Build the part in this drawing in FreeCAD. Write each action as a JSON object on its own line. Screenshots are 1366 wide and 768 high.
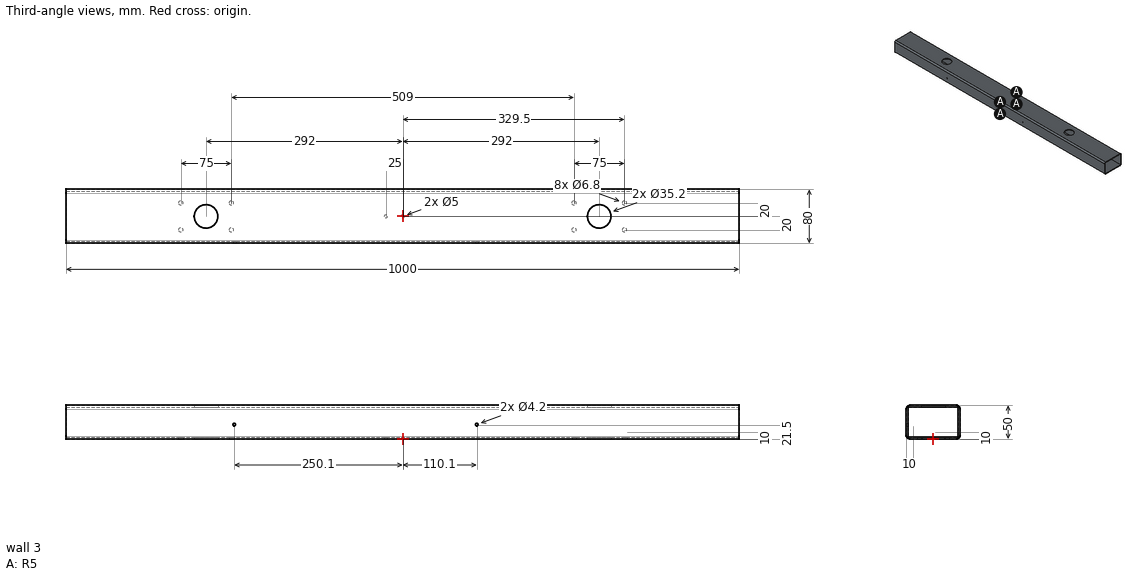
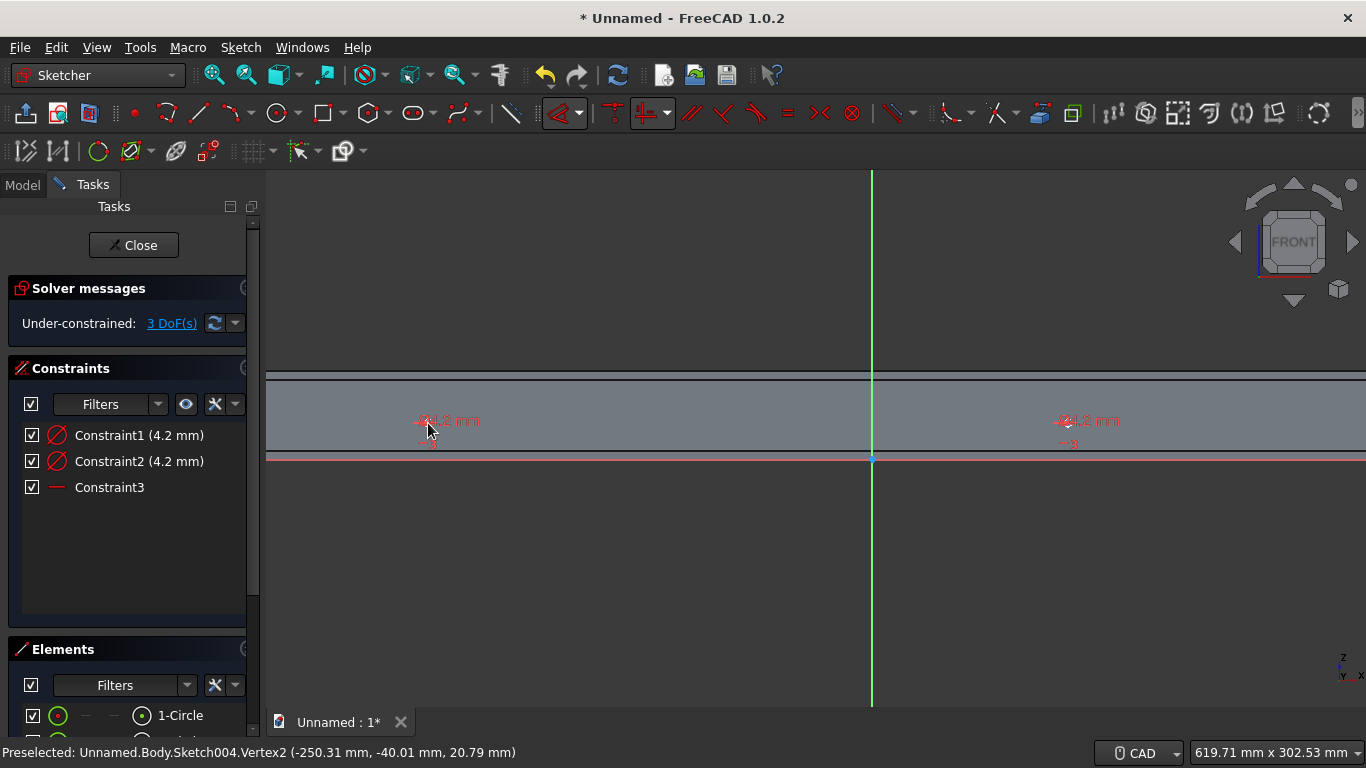
{"action": "left_click", "coordinate": [1068, 423]}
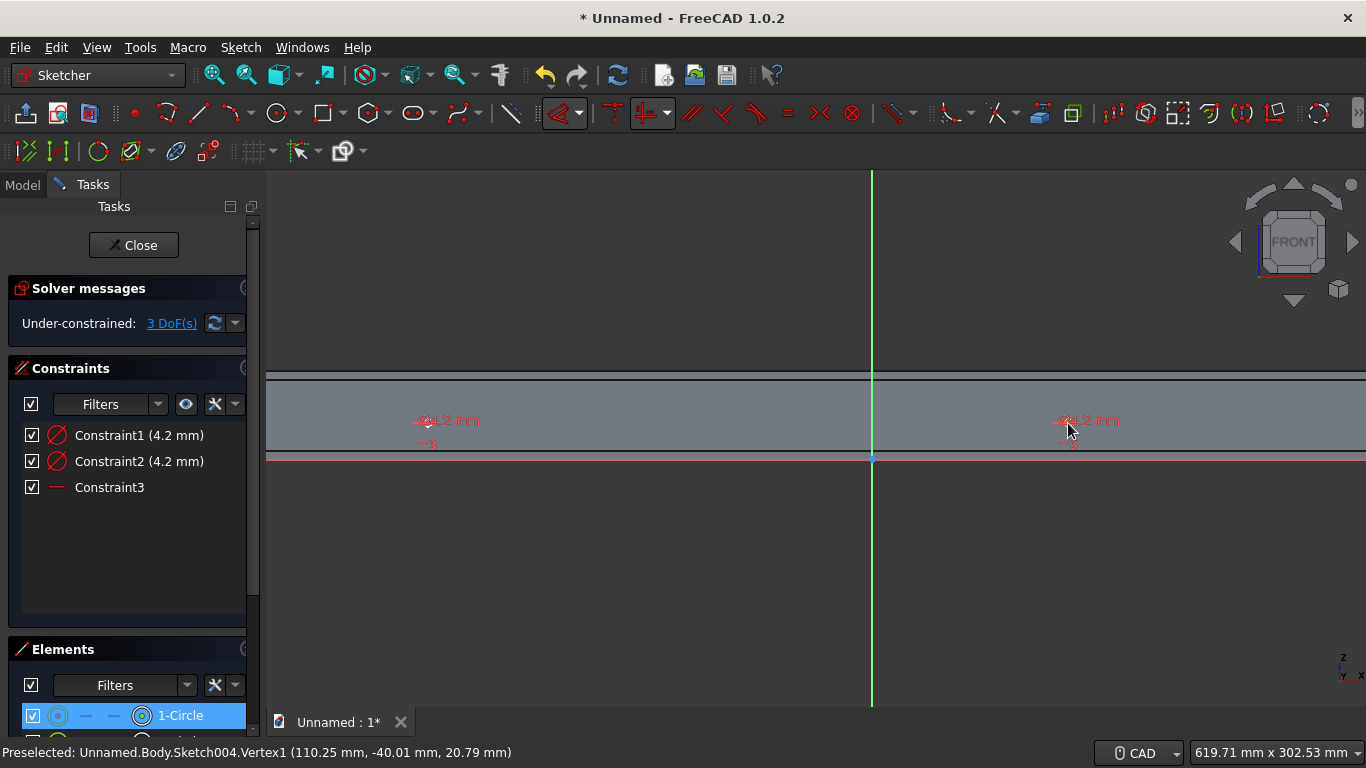
{"action": "left_click", "coordinate": [582, 114]}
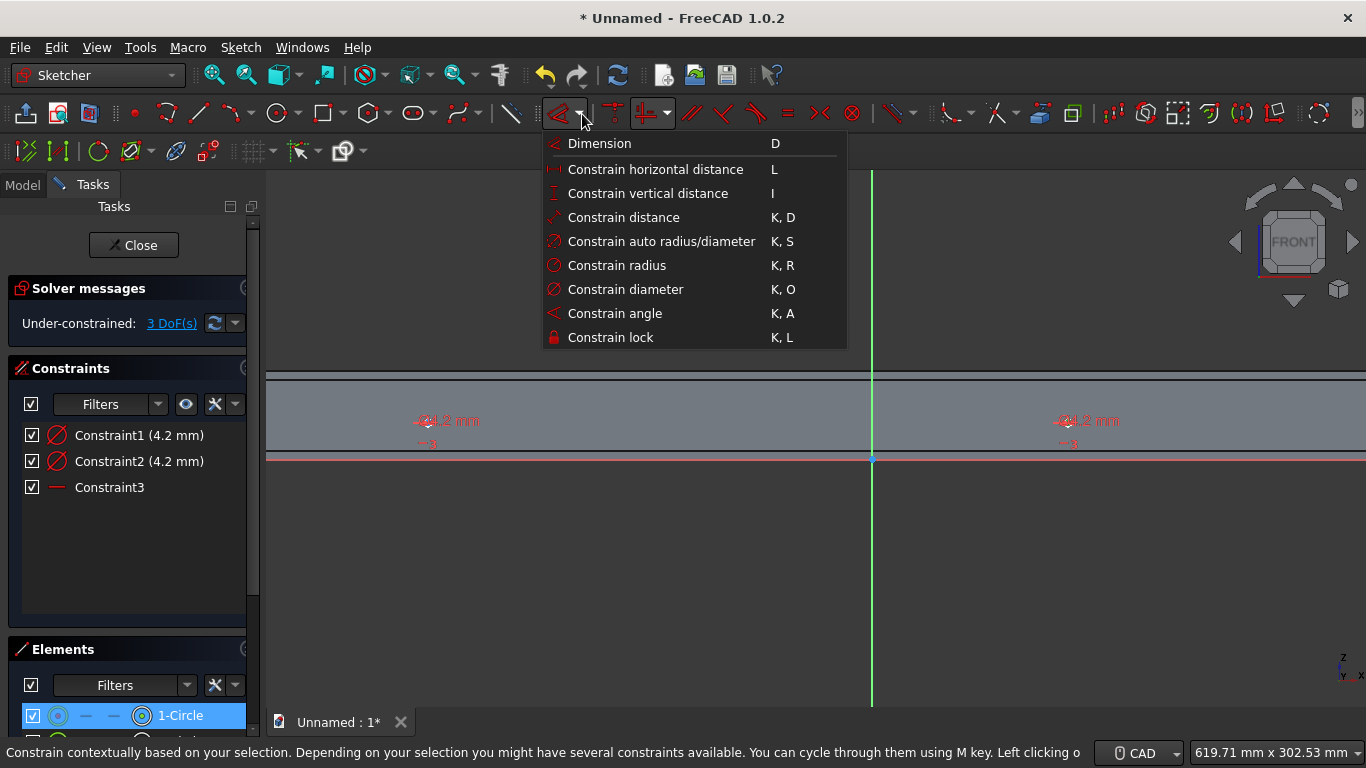
{"action": "left_click", "coordinate": [695, 193]}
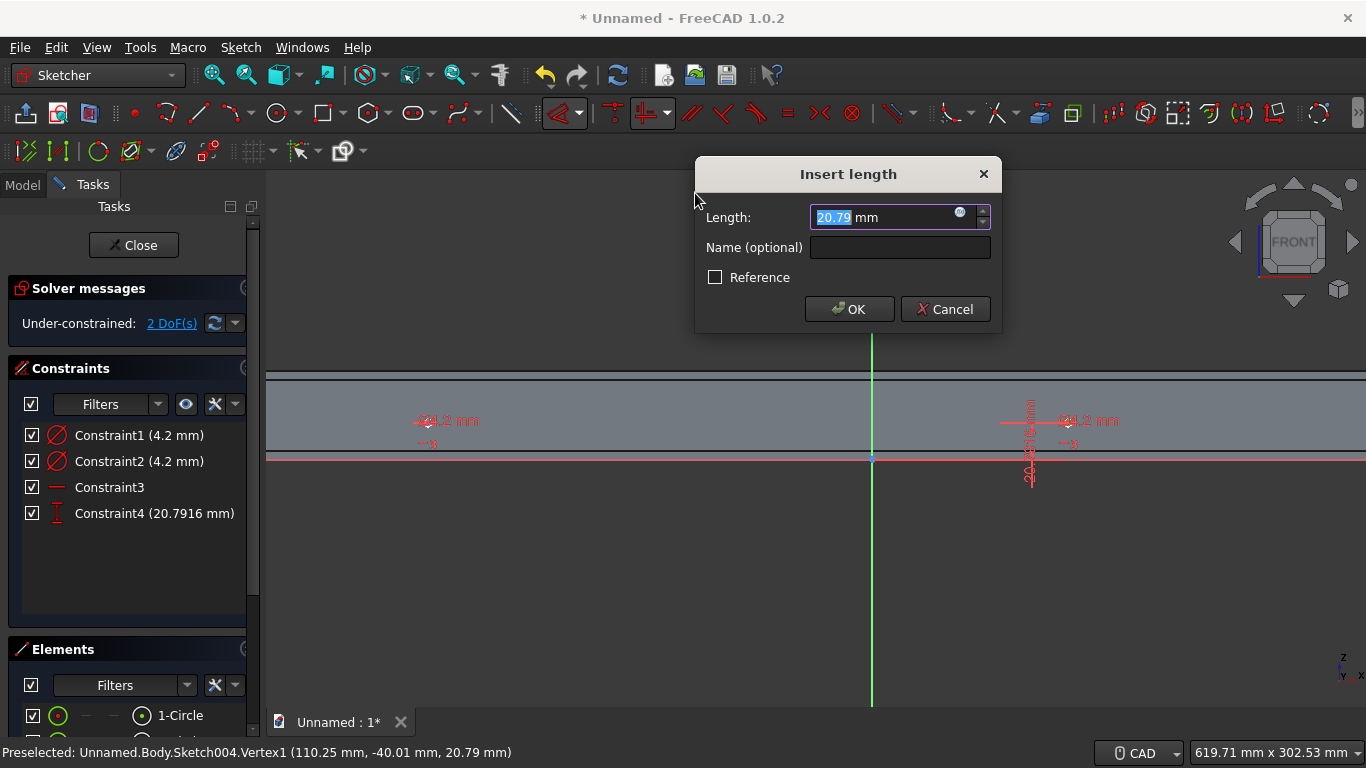
{"action": "type", "text": "21.5"}
{"action": "key", "text": "Return"}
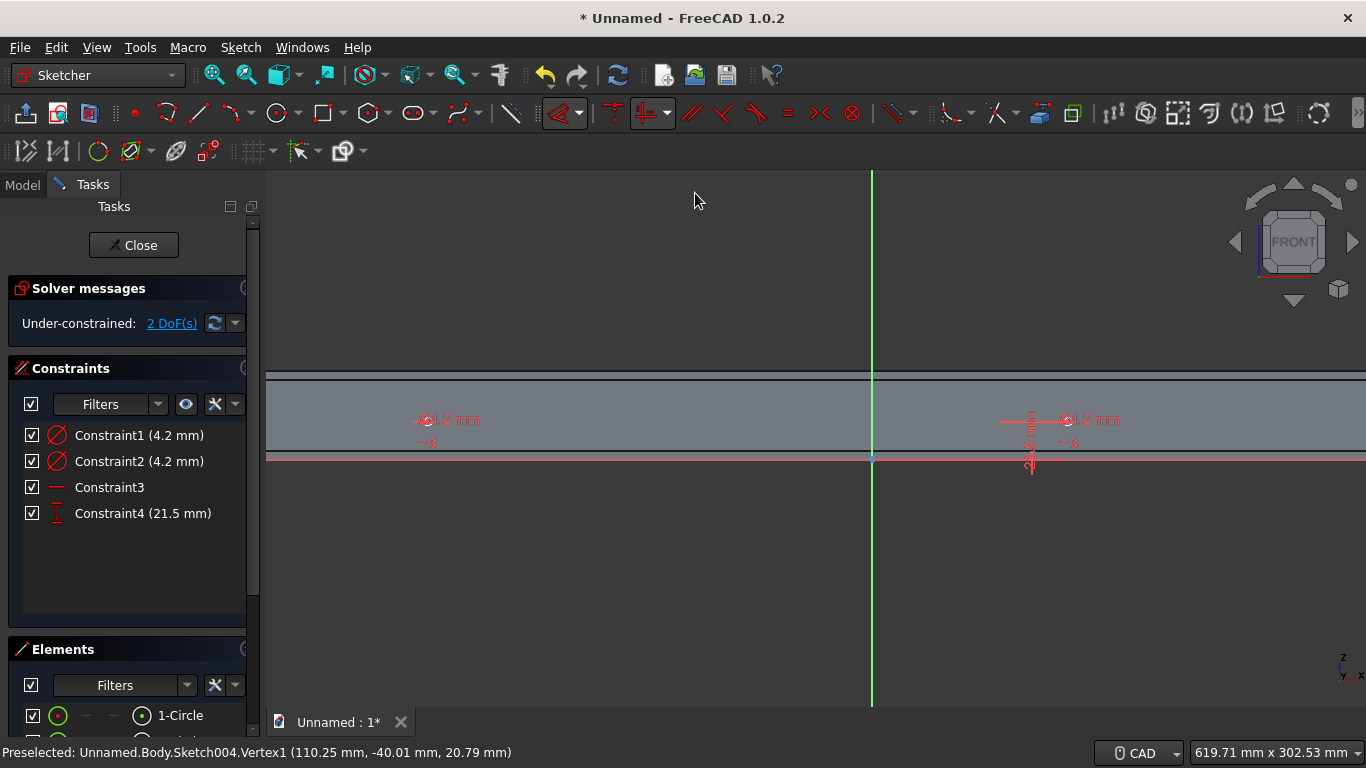
{"action": "left_click", "coordinate": [1068, 422]}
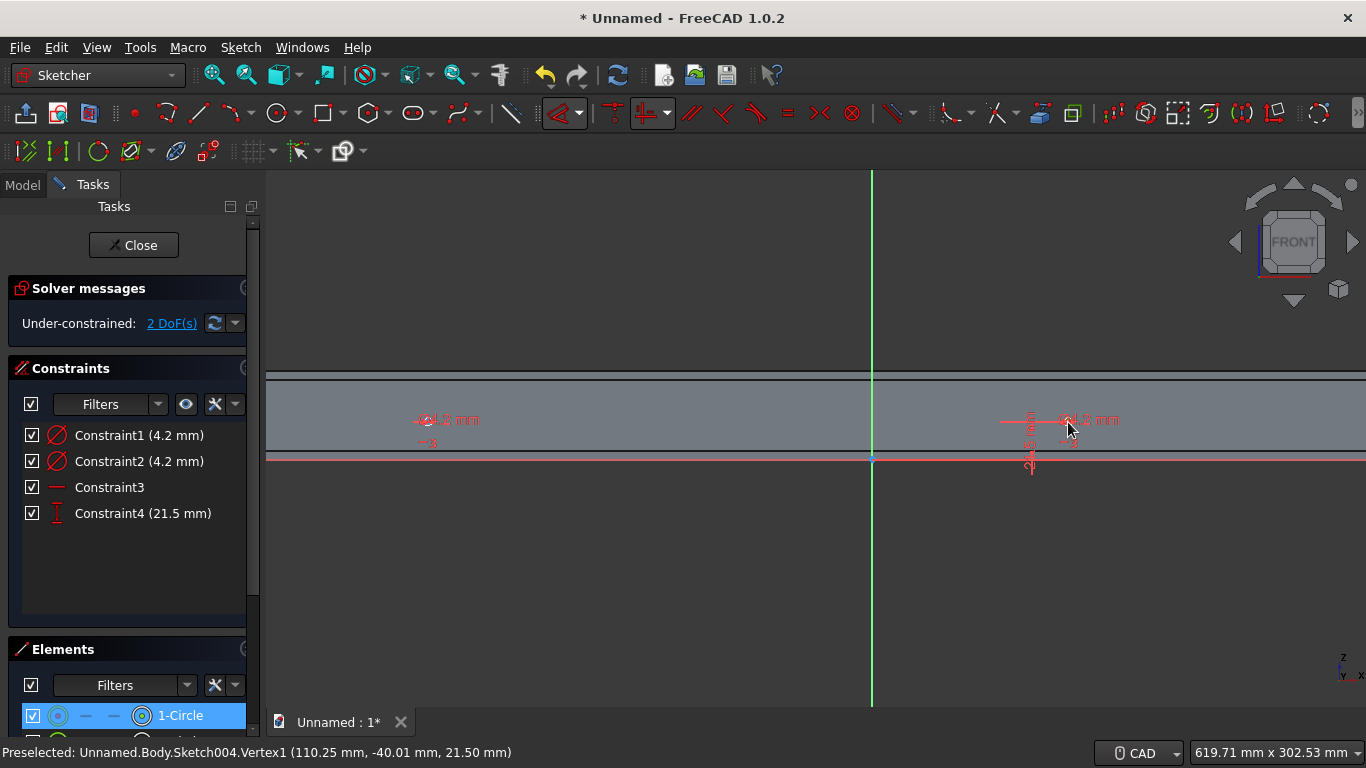
{"action": "key", "text": "l"}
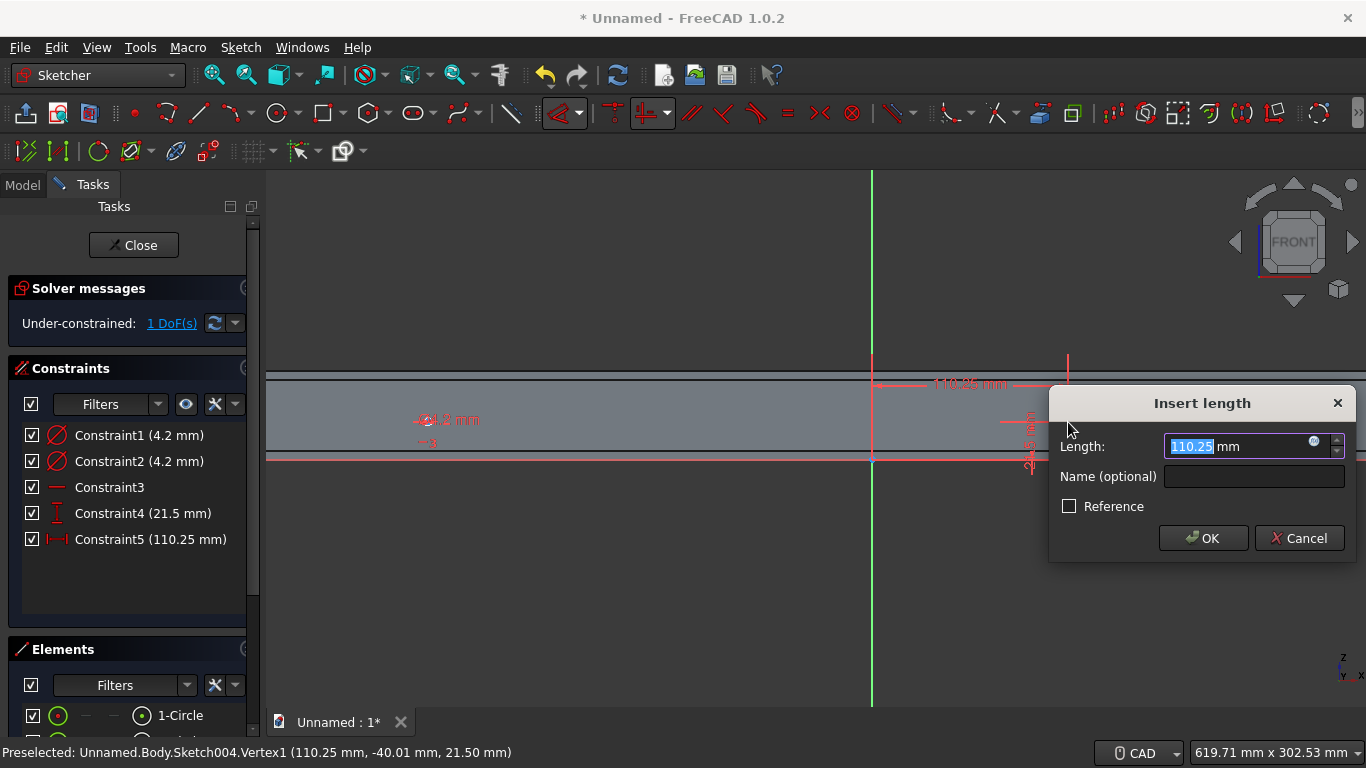
{"action": "type", "text": "110.1"}
{"action": "key", "text": "Return"}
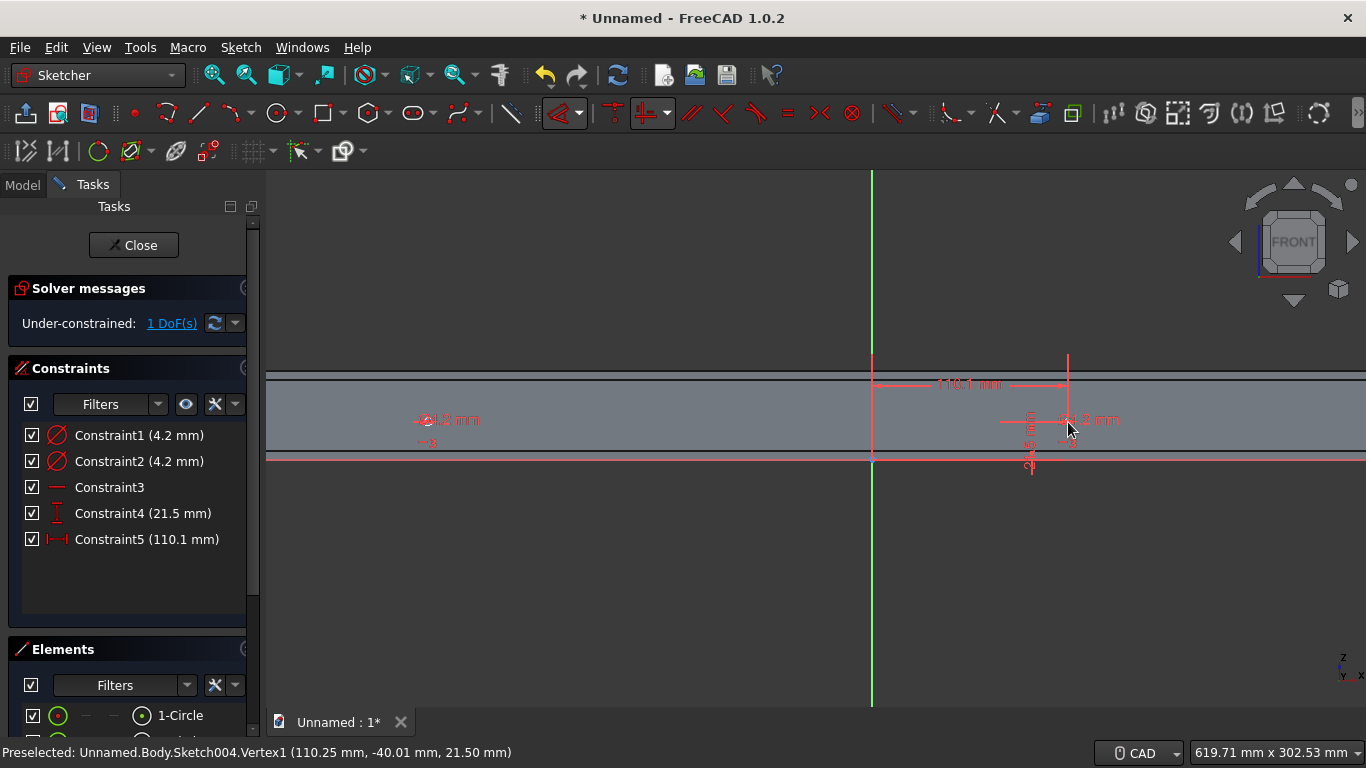
{"action": "left_click", "coordinate": [428, 422]}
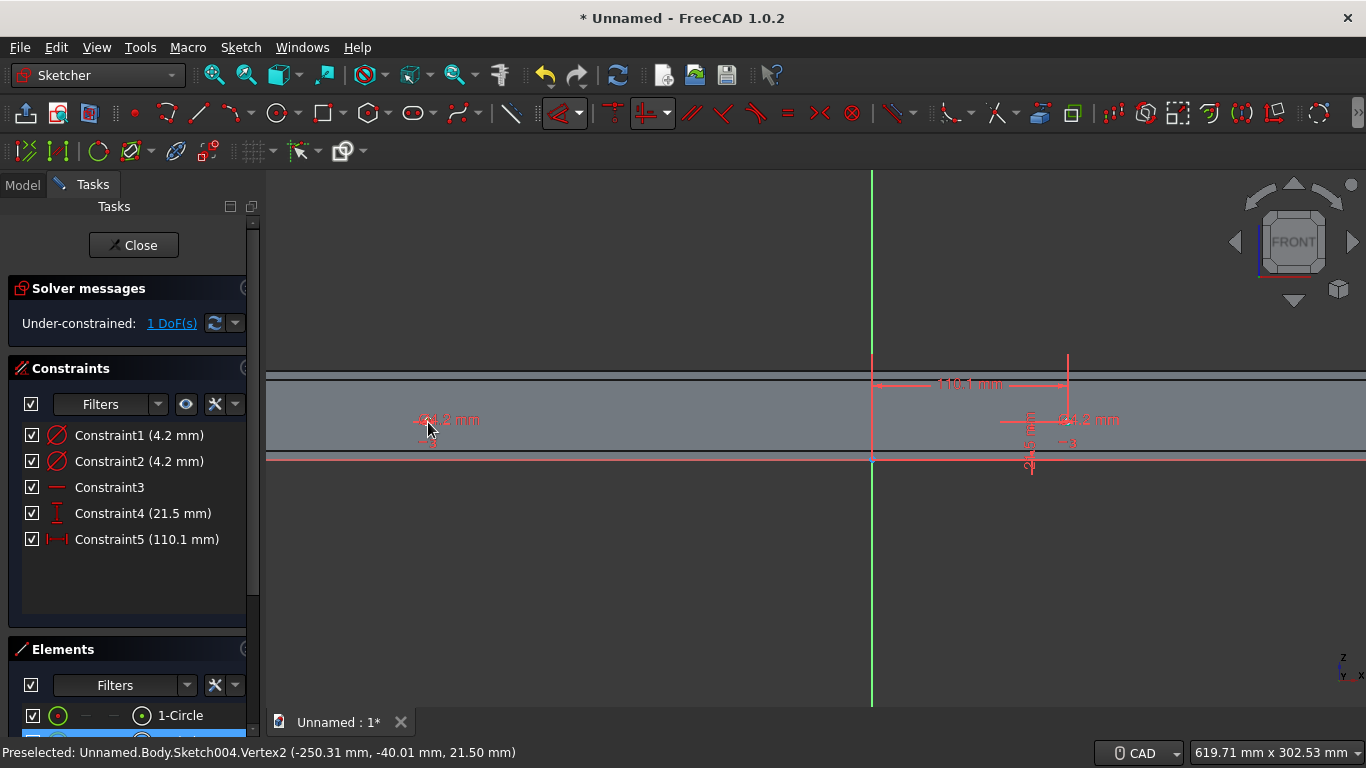
{"action": "left_click", "coordinate": [582, 114]}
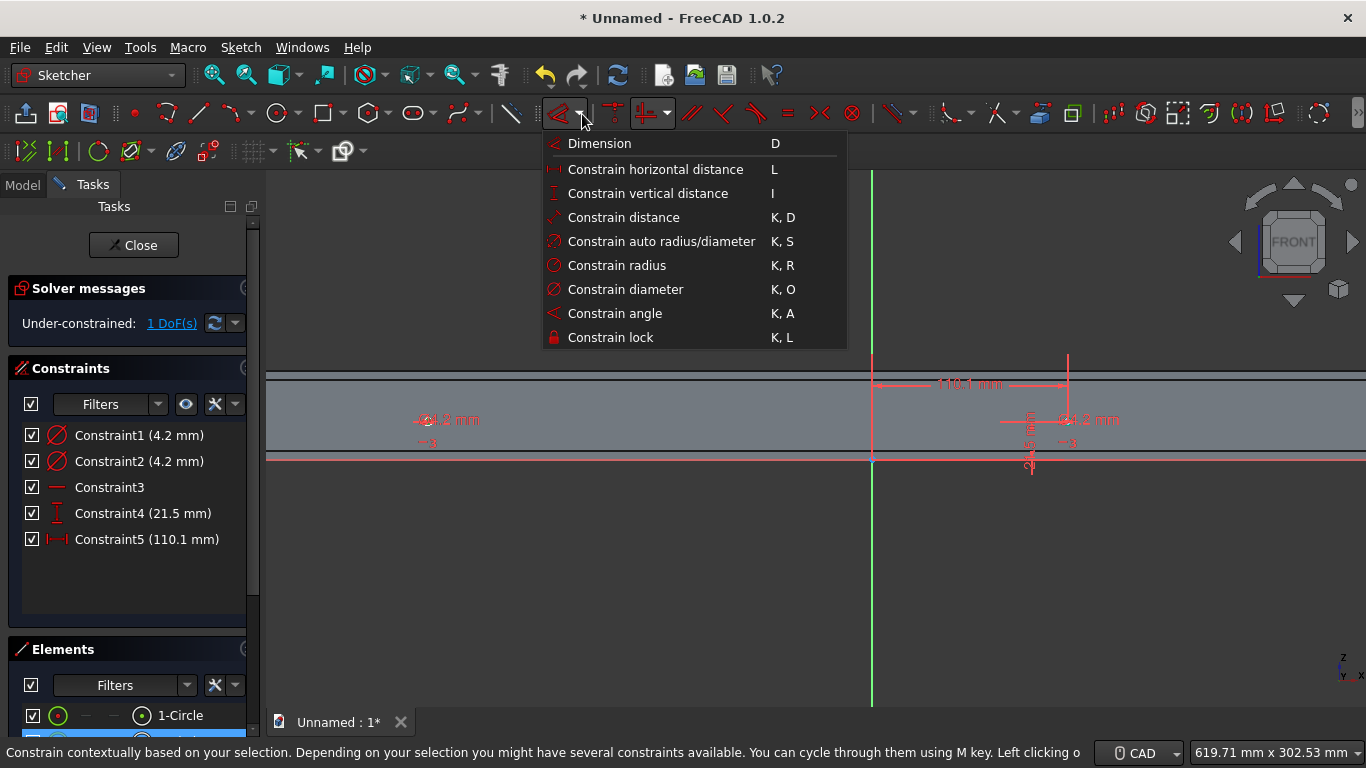
{"action": "left_click", "coordinate": [695, 169]}